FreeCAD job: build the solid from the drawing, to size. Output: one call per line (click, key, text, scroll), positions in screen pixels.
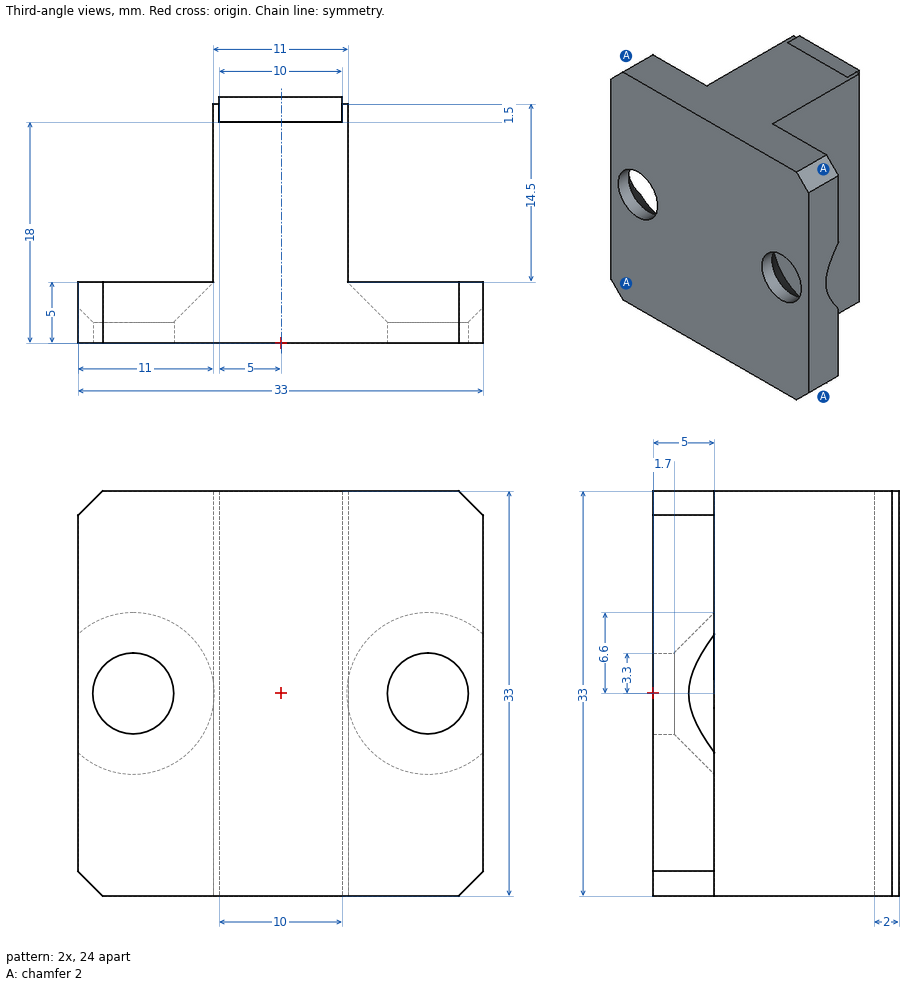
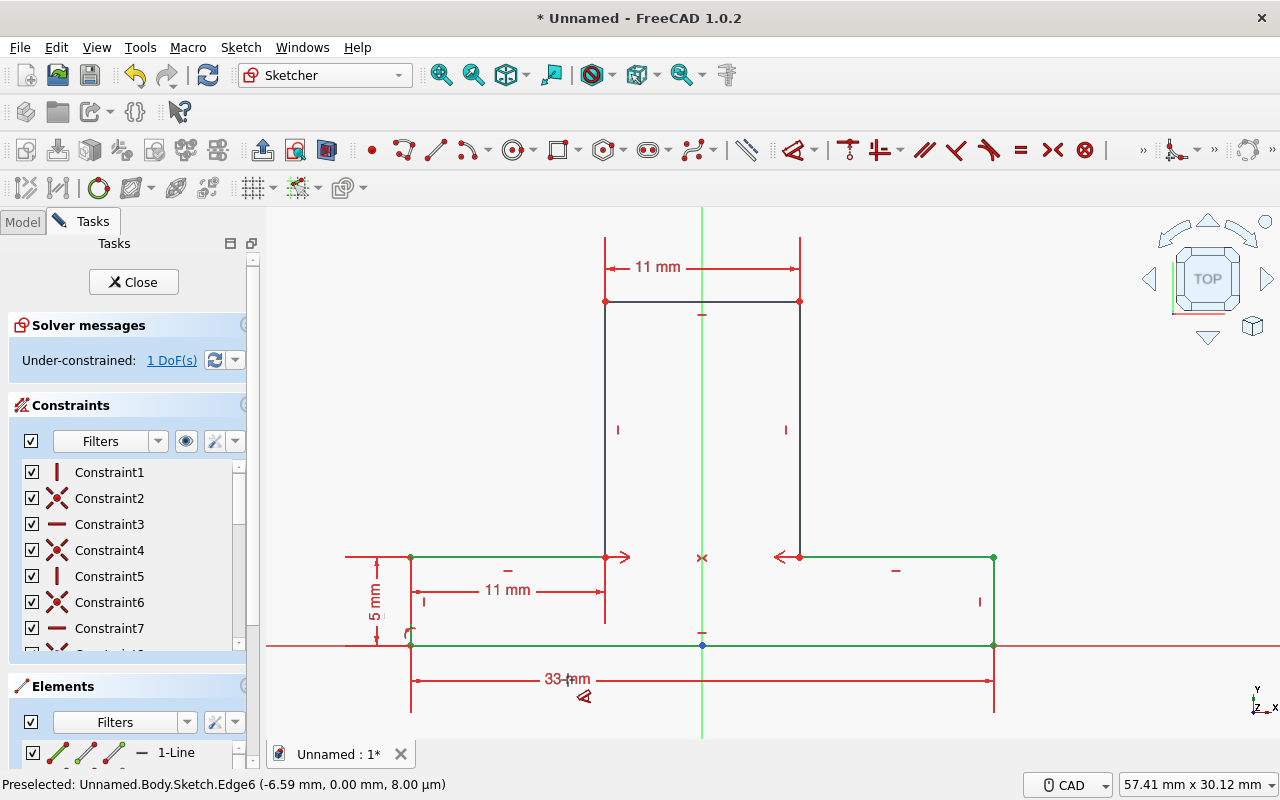
click(800, 481)
click(834, 429)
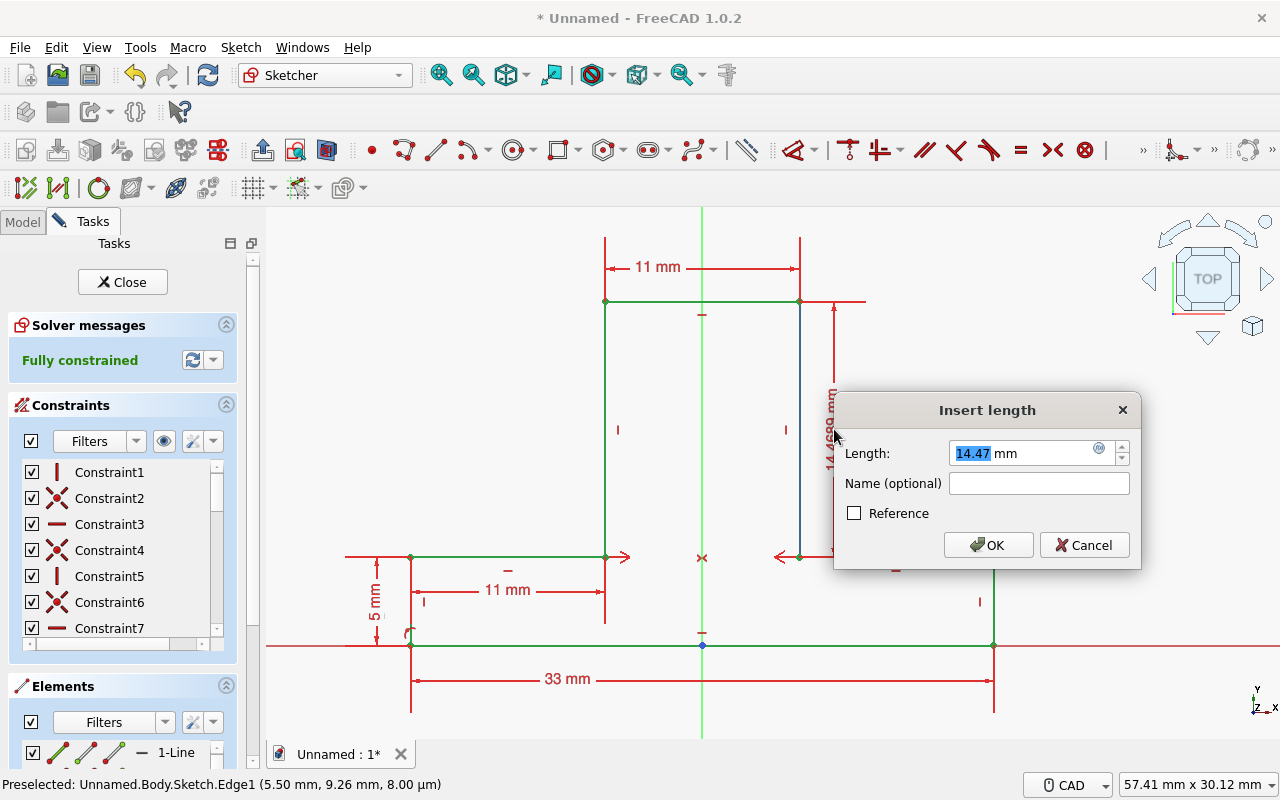
text(14.5)
key(Return)
key(Escape)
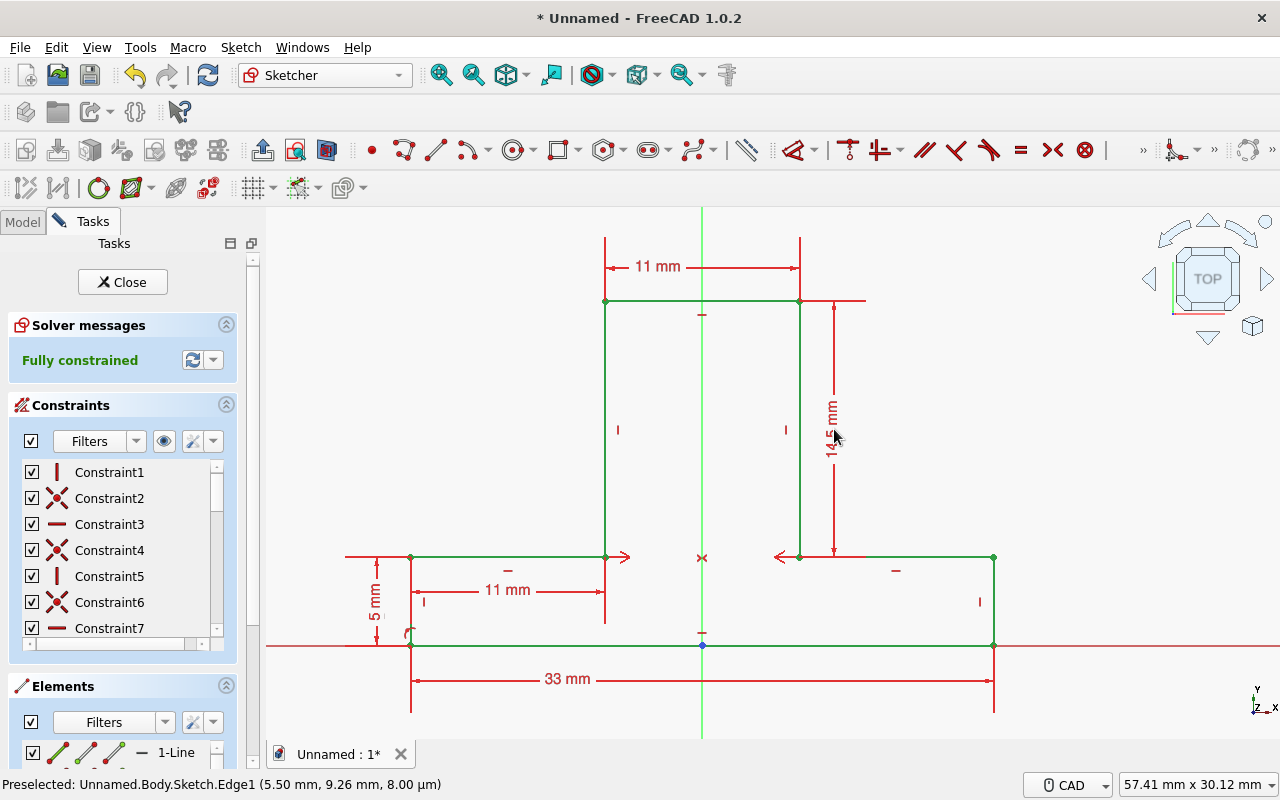
click(123, 282)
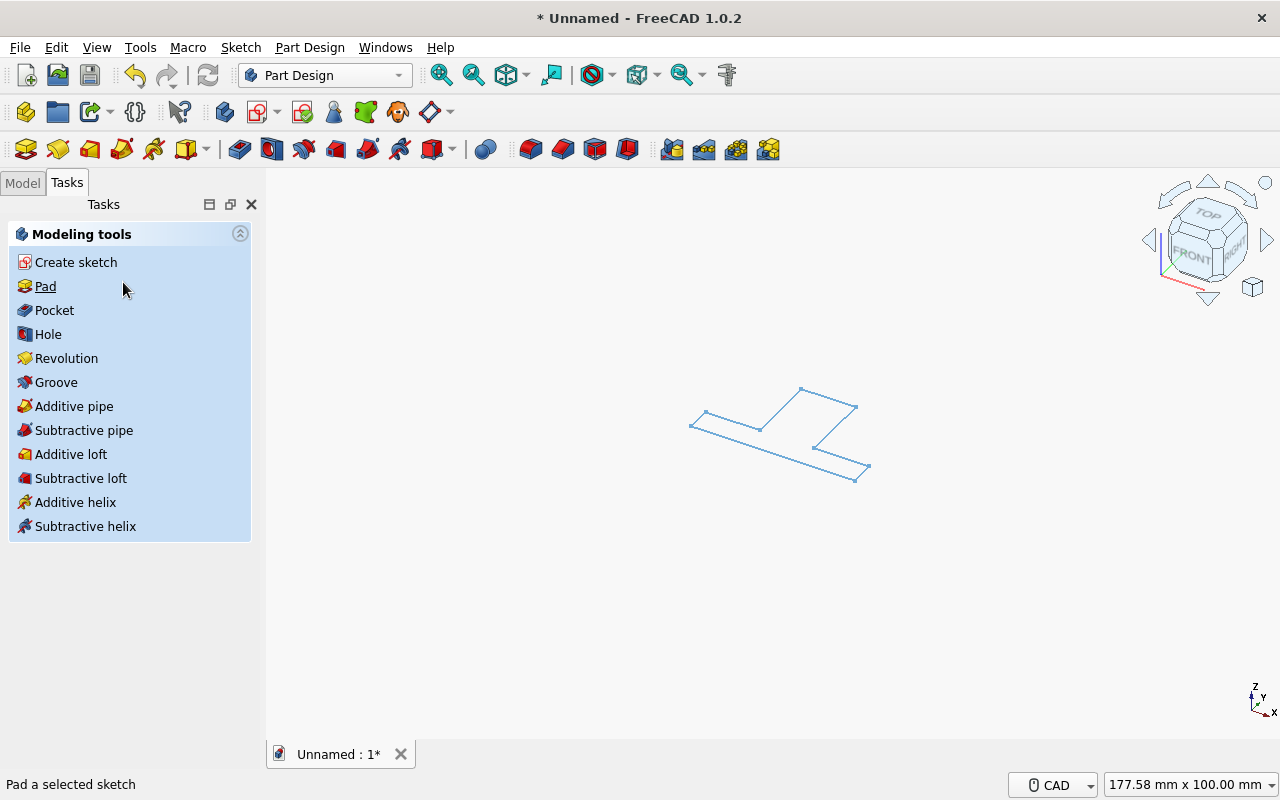
click(26, 150)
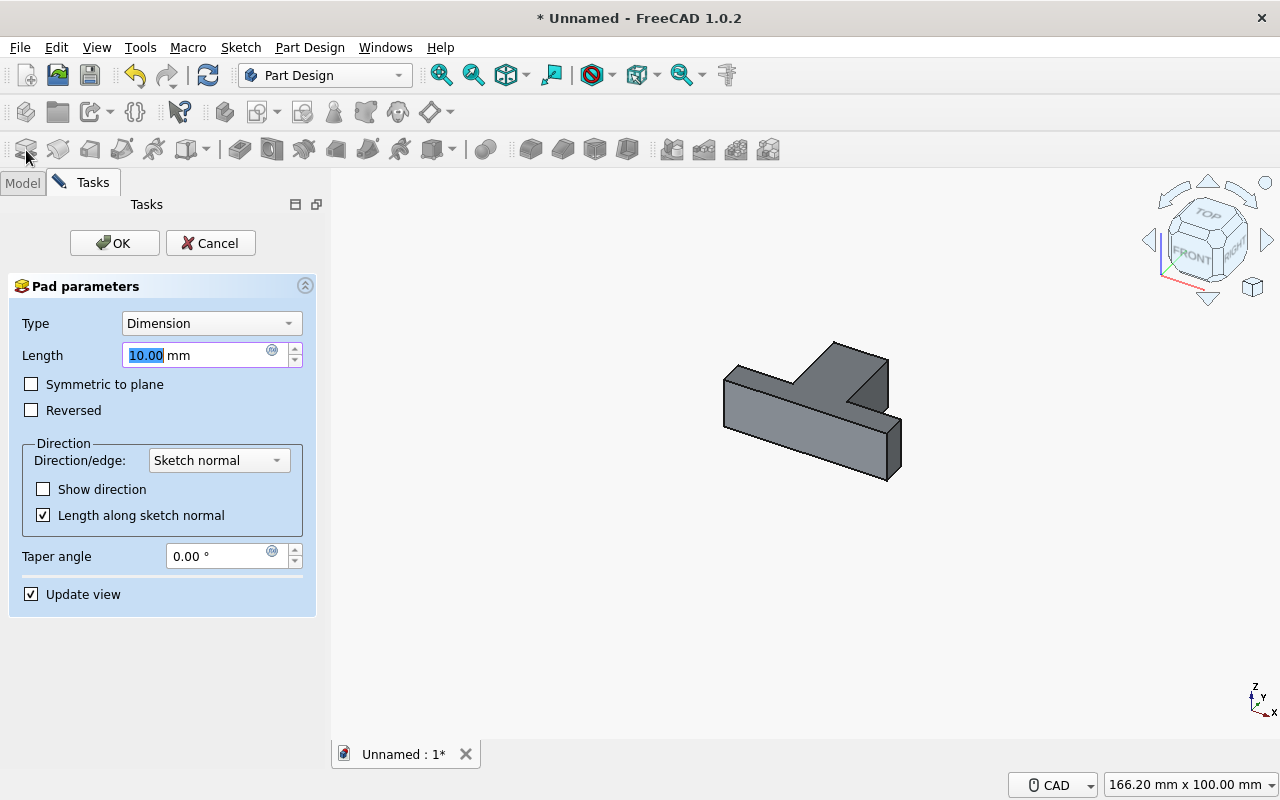
text(33)
key(Tab)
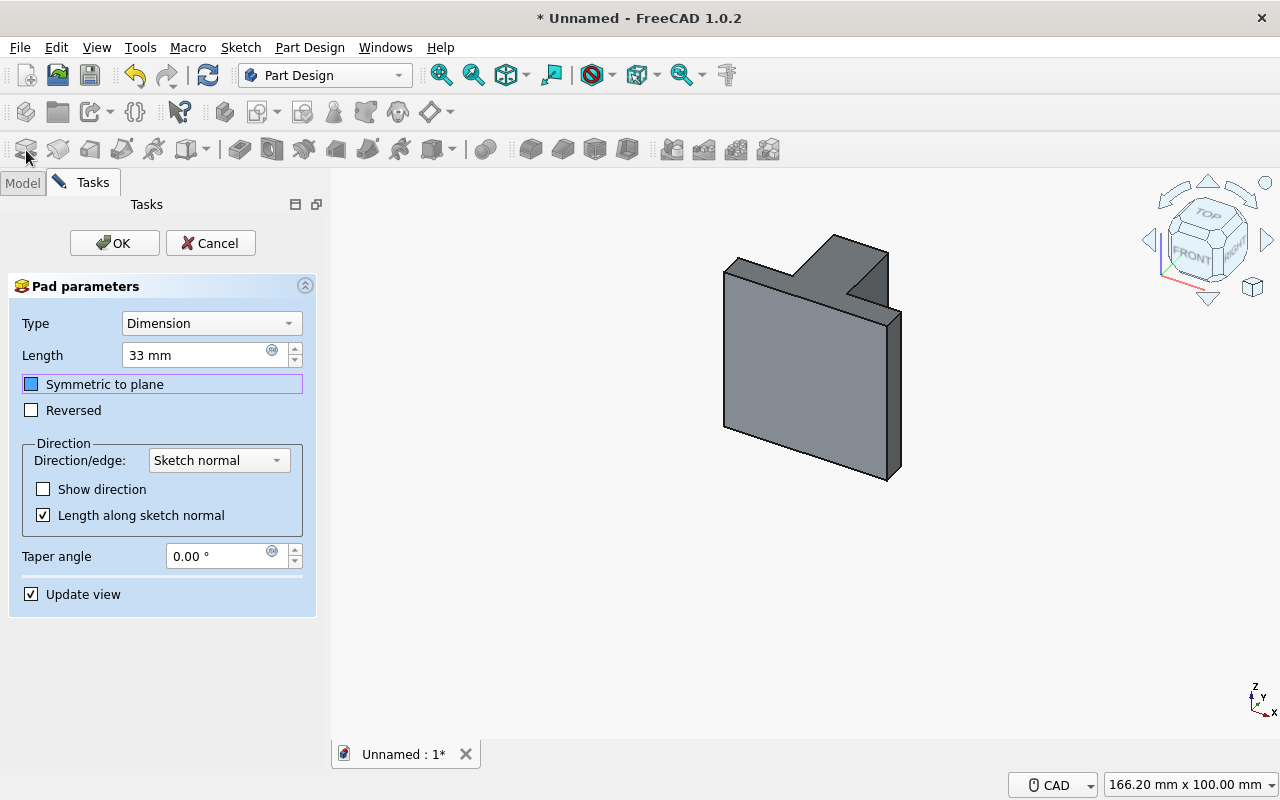
click(30, 384)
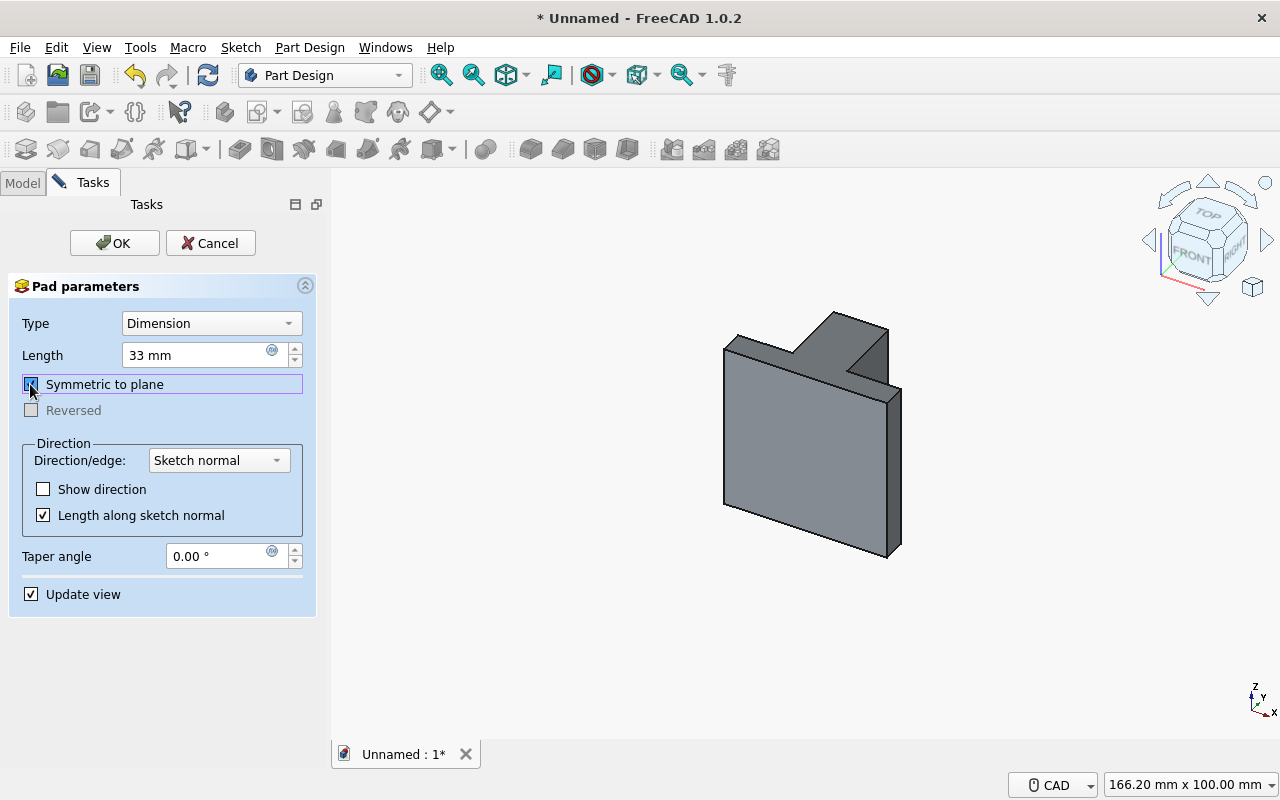
click(115, 243)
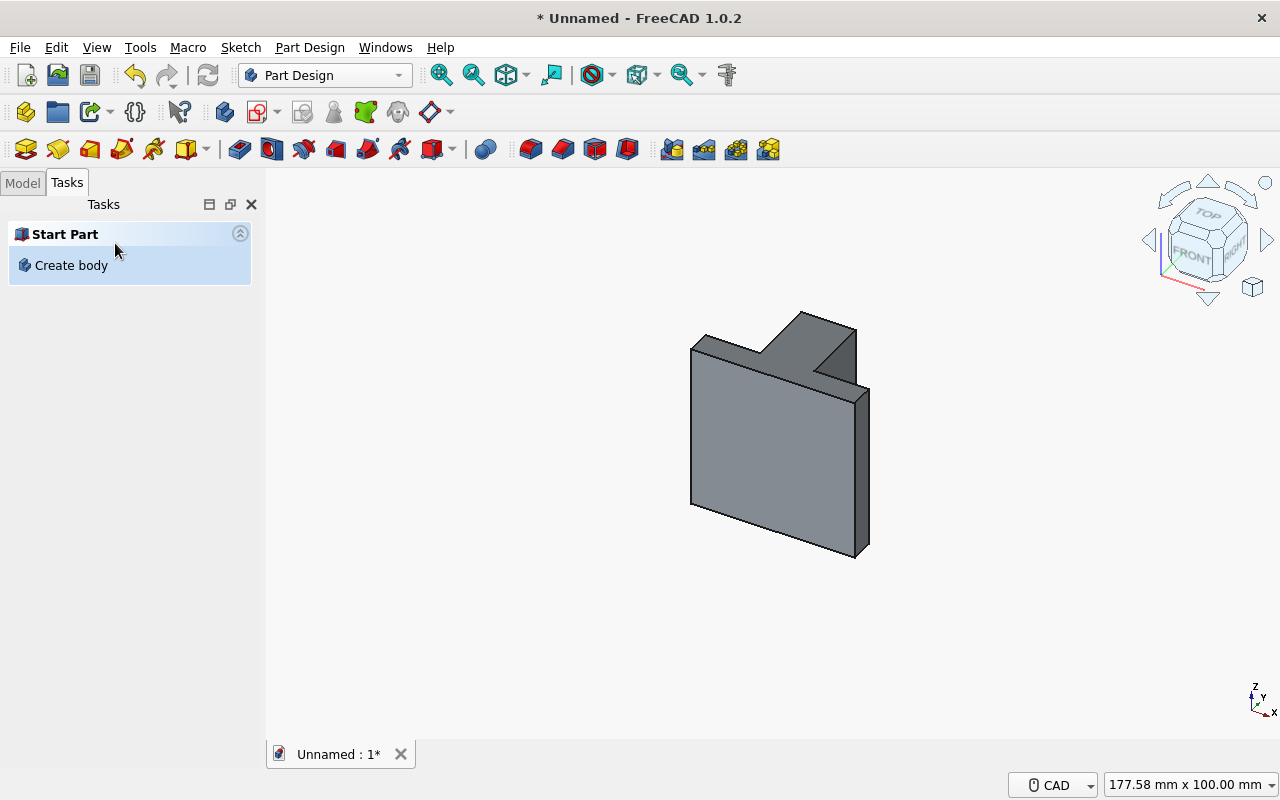
click(809, 340)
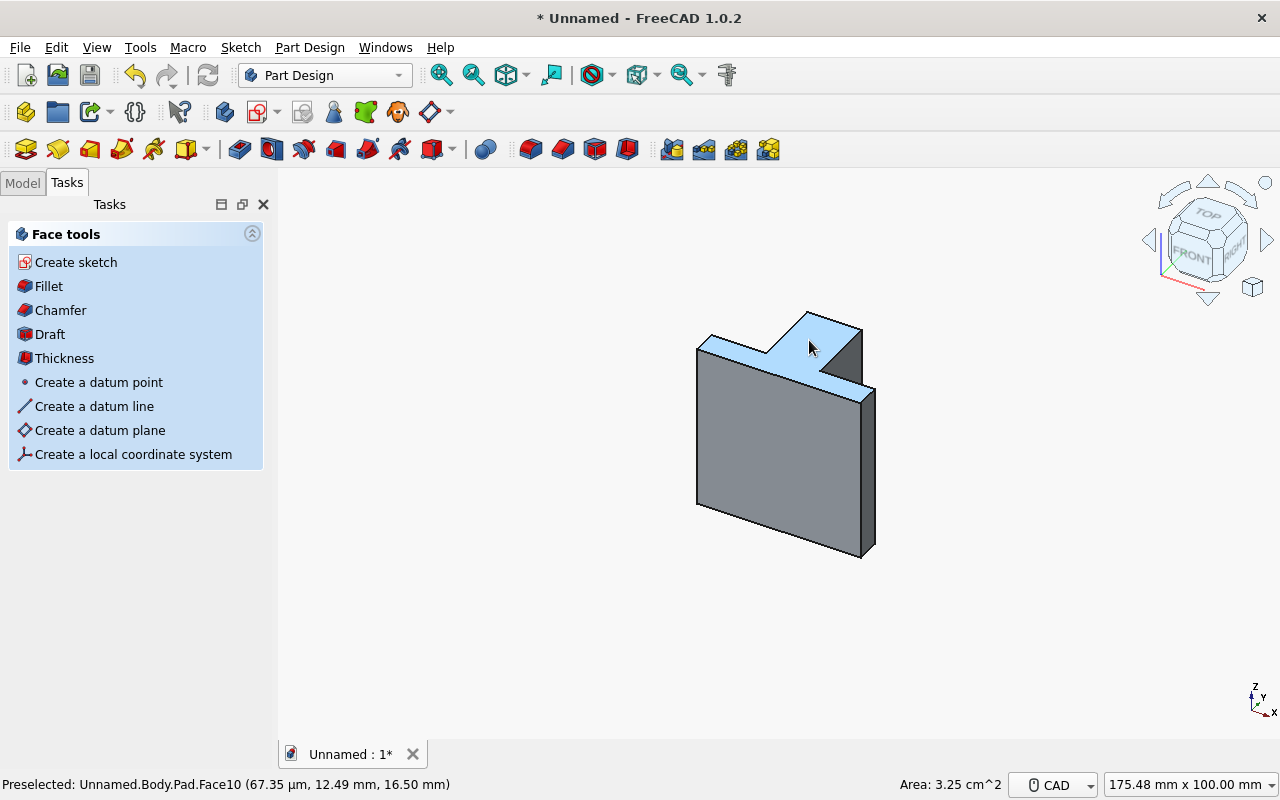
click(258, 112)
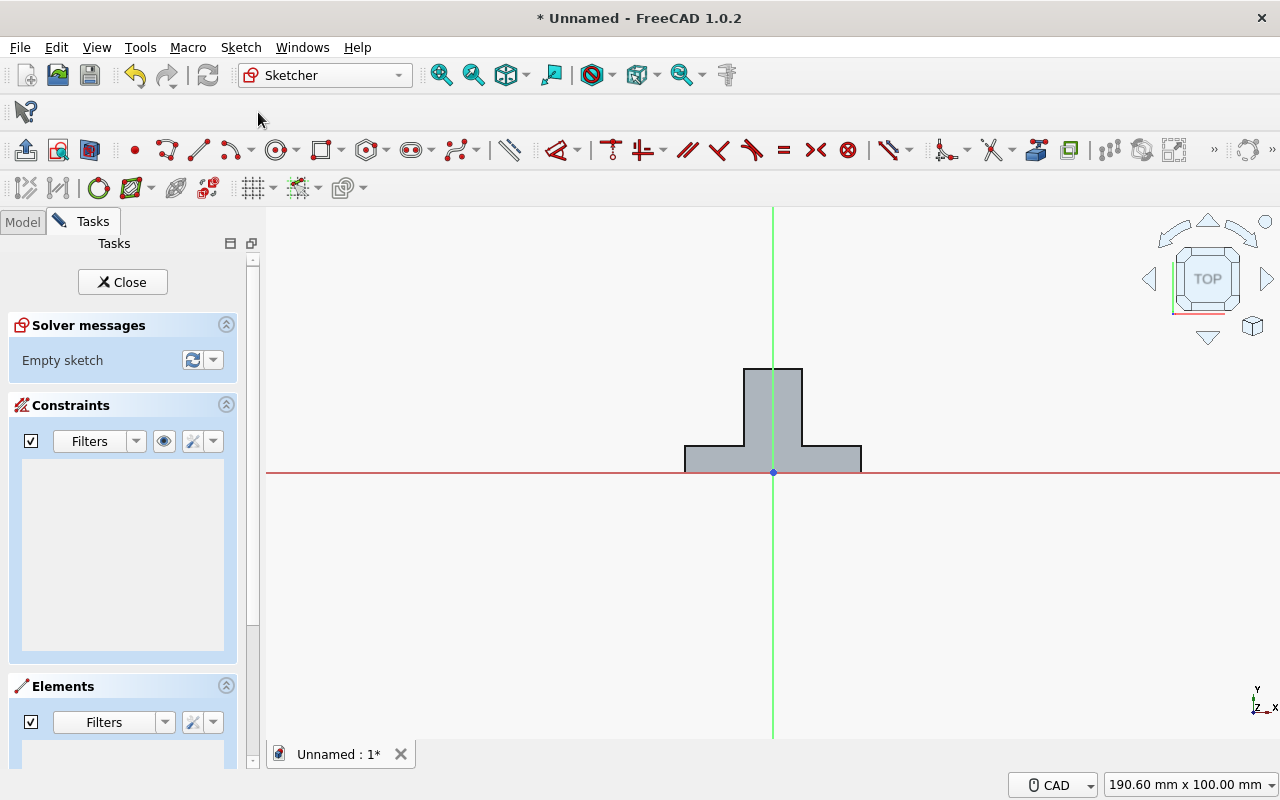
scroll(803, 399, up, 6)